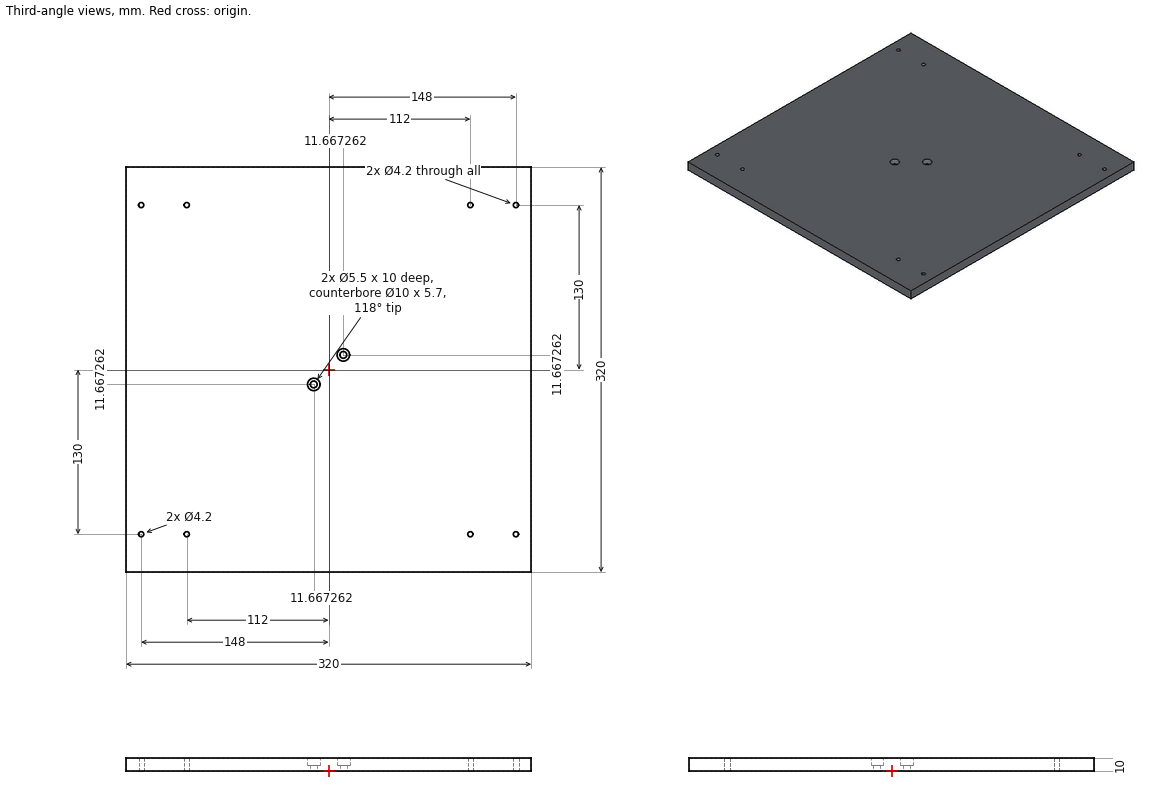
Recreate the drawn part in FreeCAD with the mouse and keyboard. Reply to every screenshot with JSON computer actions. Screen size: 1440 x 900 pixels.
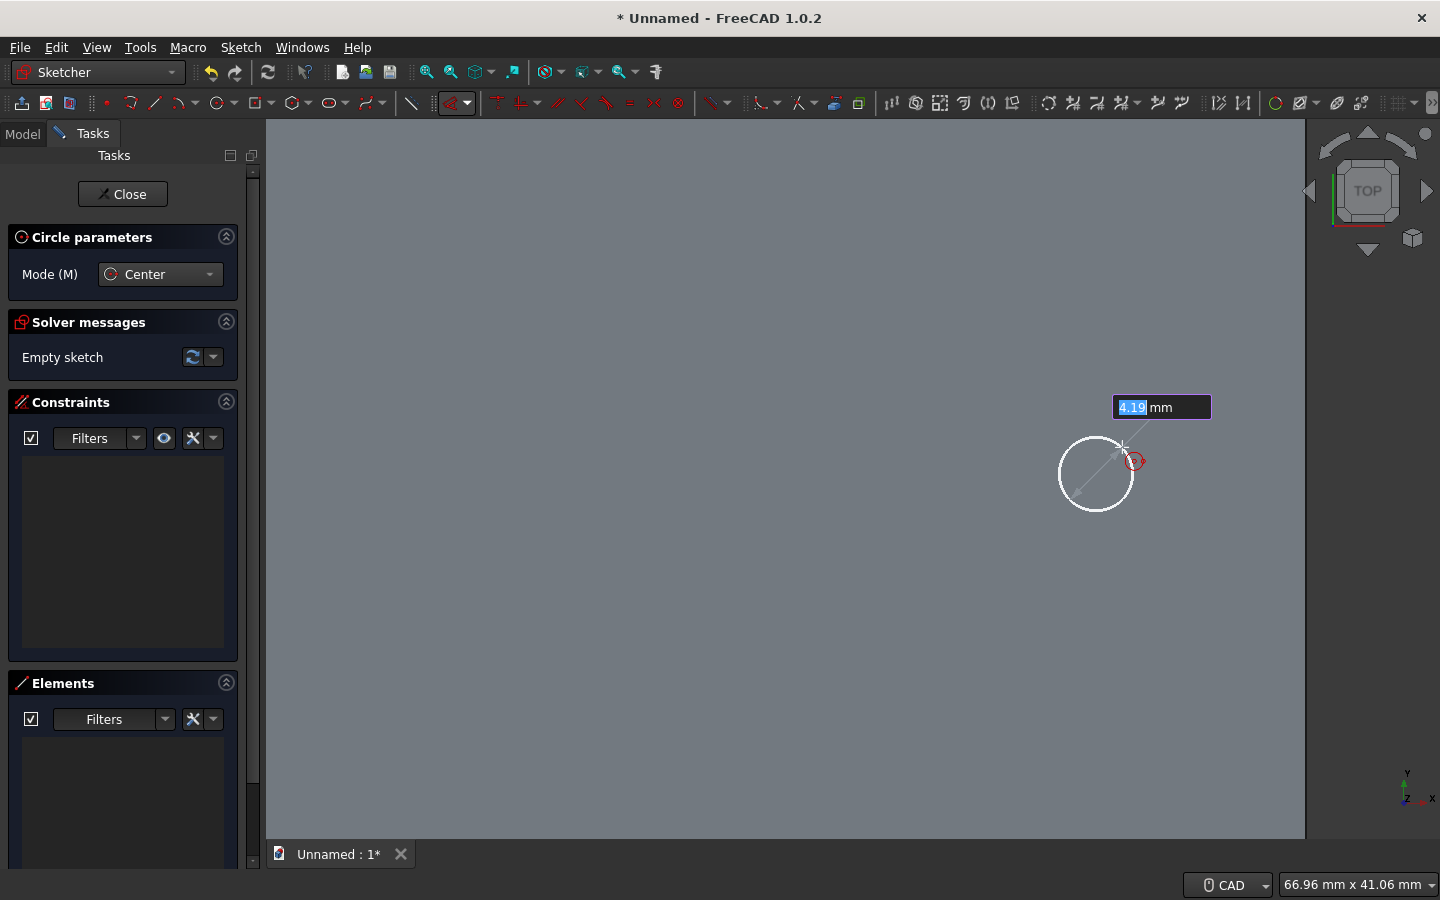
{"action": "type", "text": "4.2"}
{"action": "key", "text": "Return"}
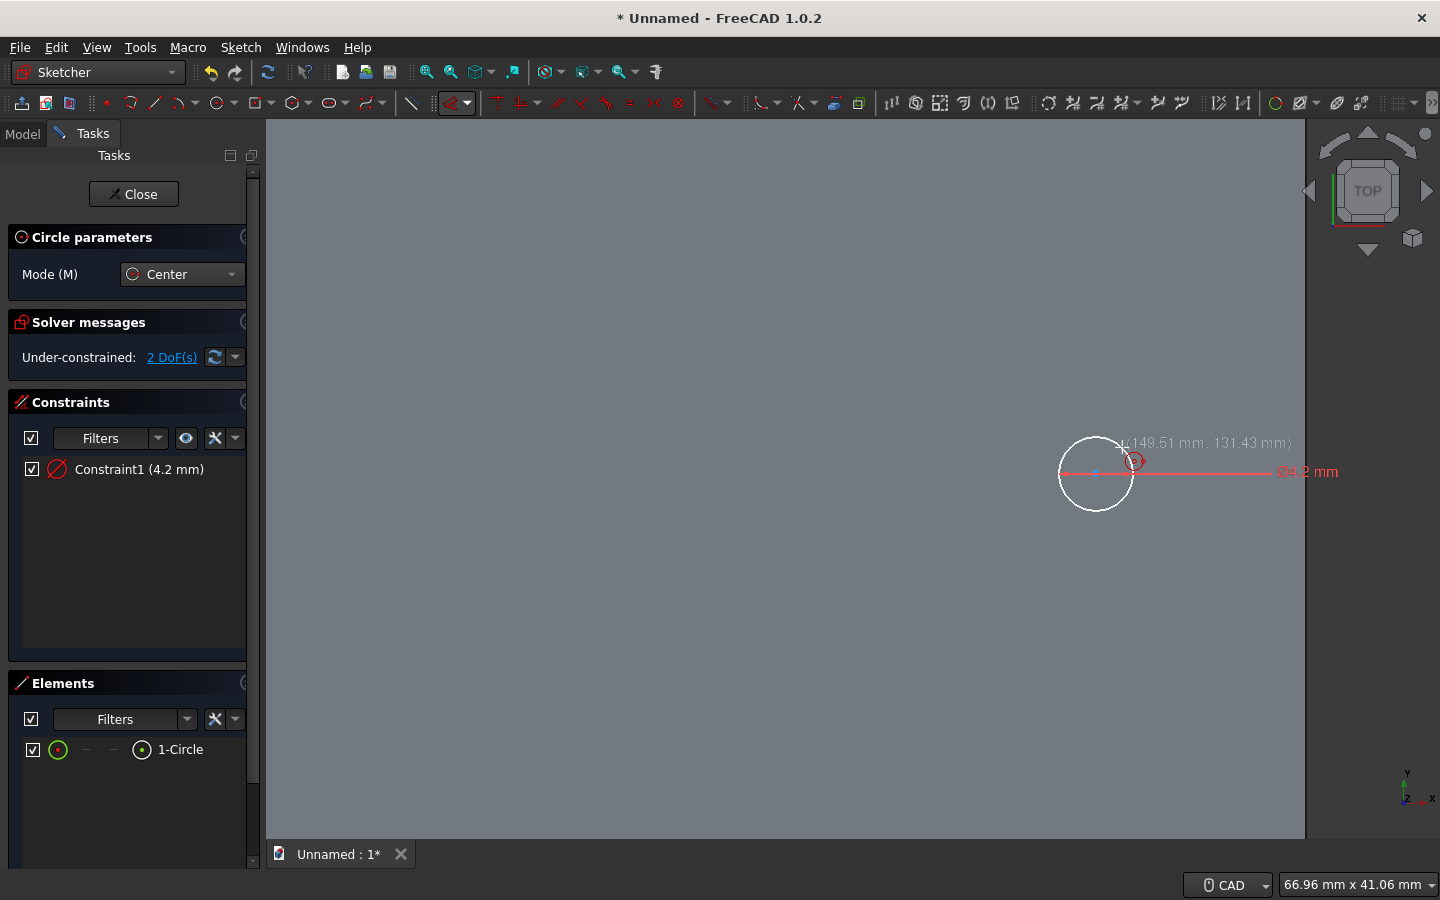
{"action": "left_click", "coordinate": [464, 473]}
{"action": "mouse_move", "coordinate": [490, 447]}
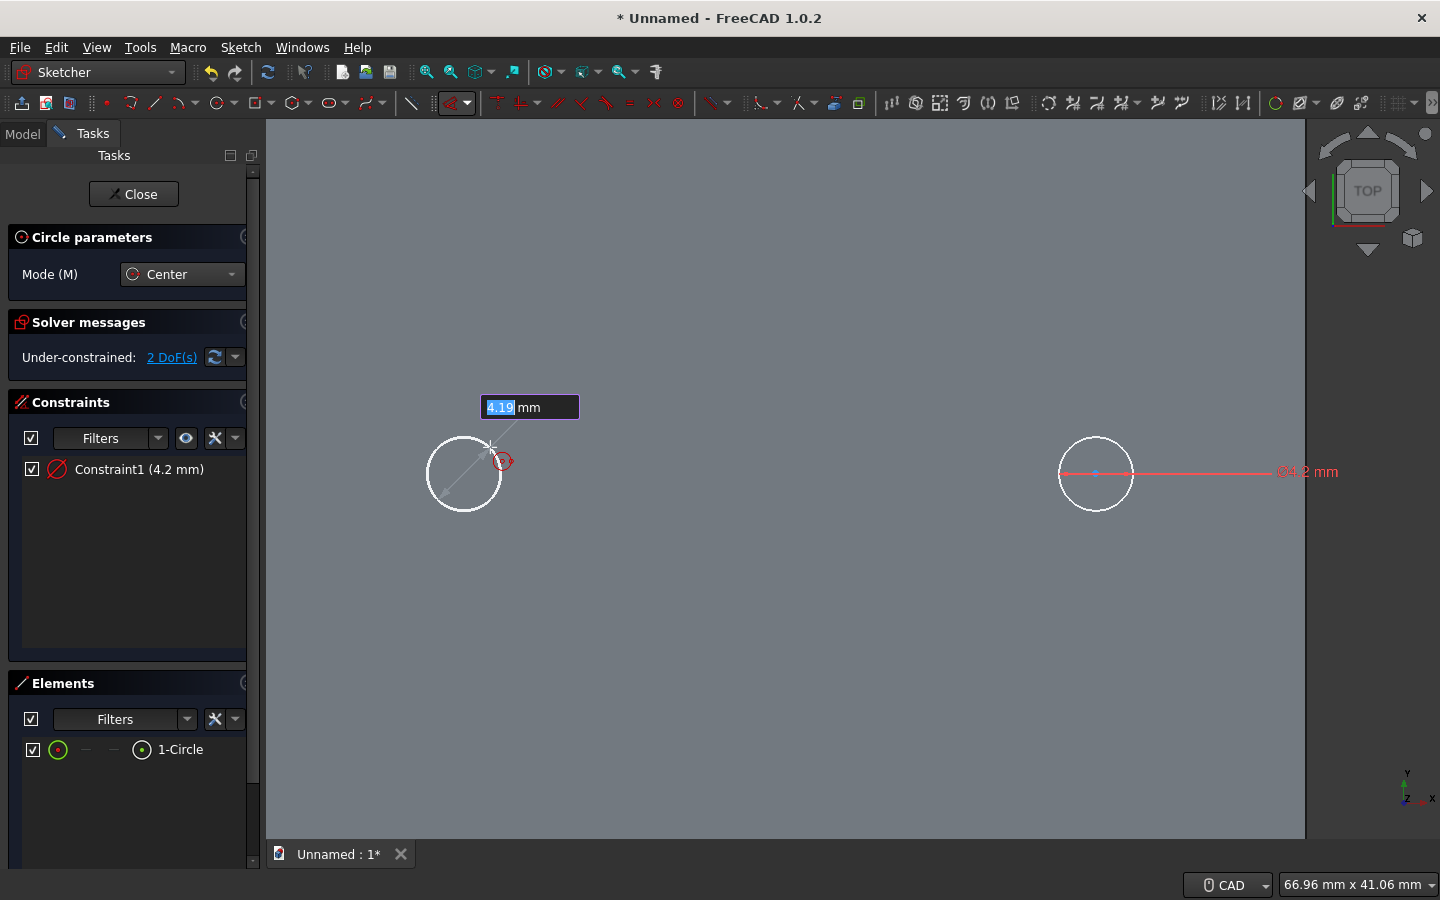
{"action": "type", "text": "4.2"}
{"action": "key", "text": "Return"}
{"action": "key", "text": "Escape"}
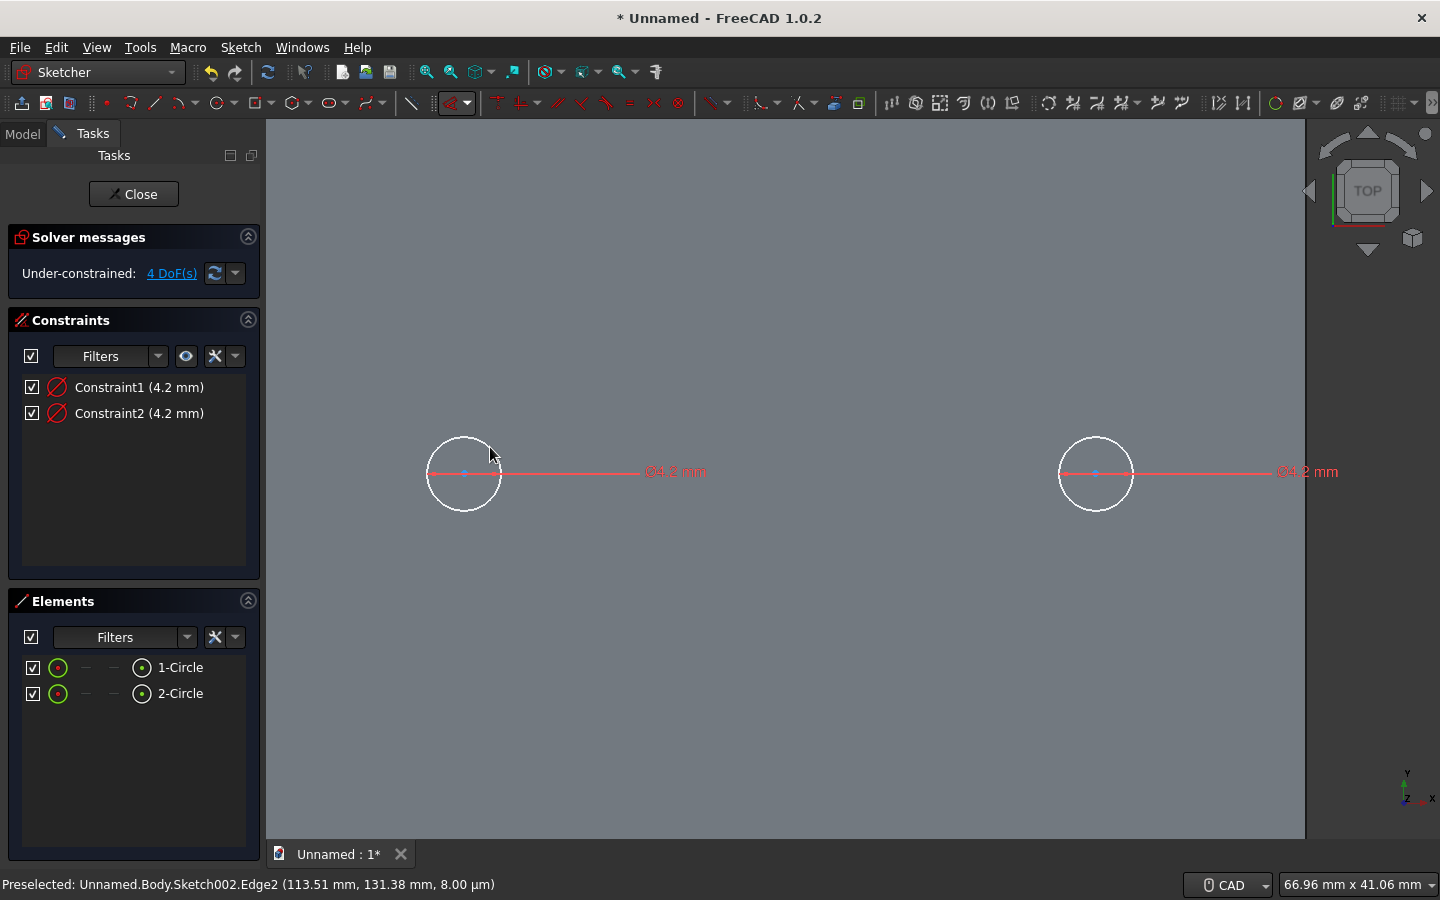
{"action": "left_click", "coordinate": [450, 104]}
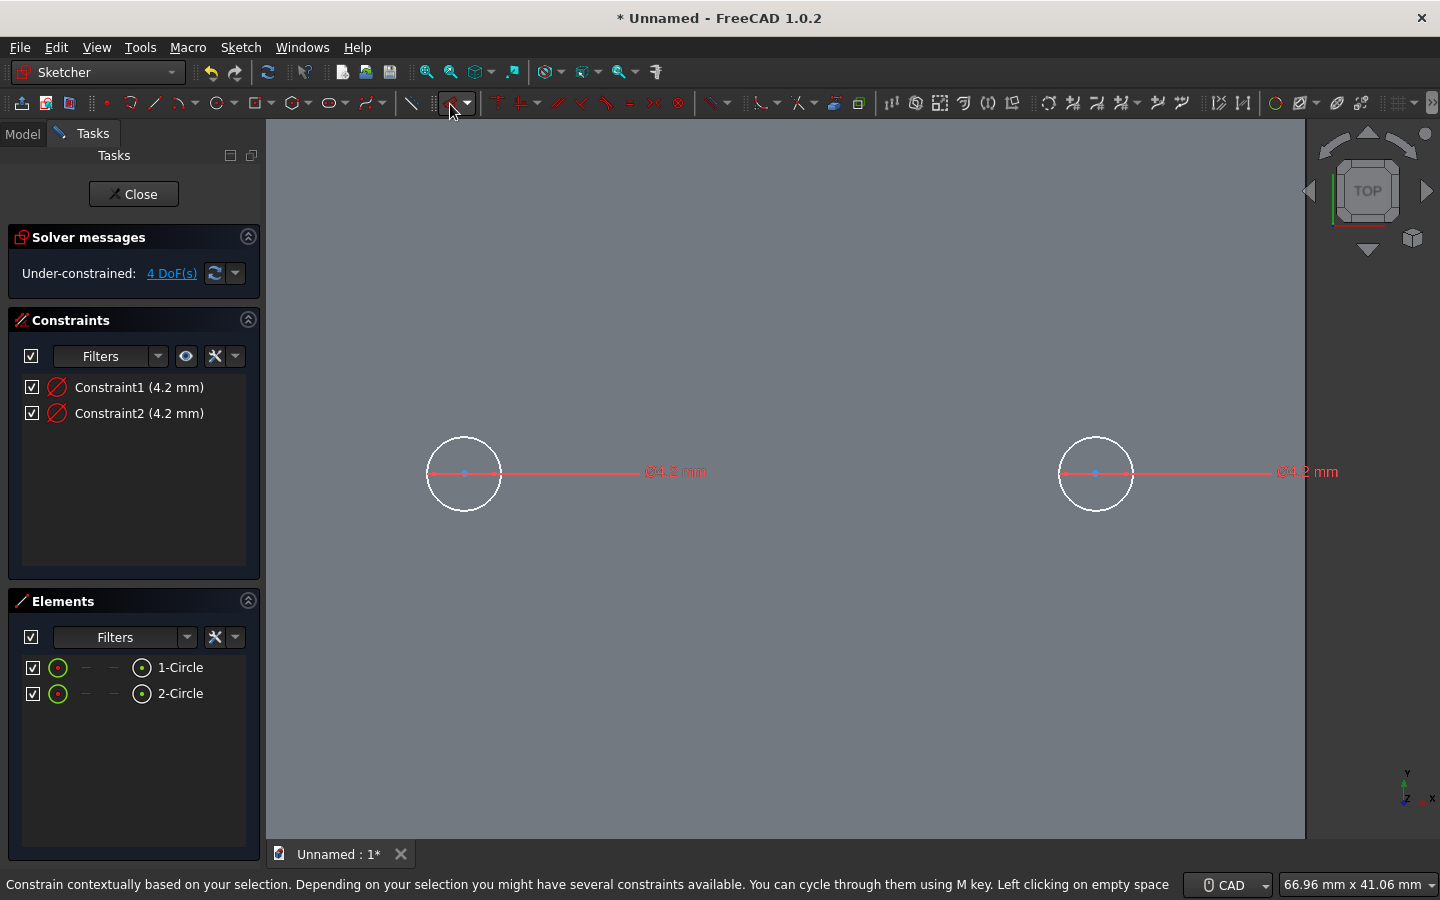
{"action": "left_click", "coordinate": [1096, 474]}
{"action": "left_click", "coordinate": [695, 440]}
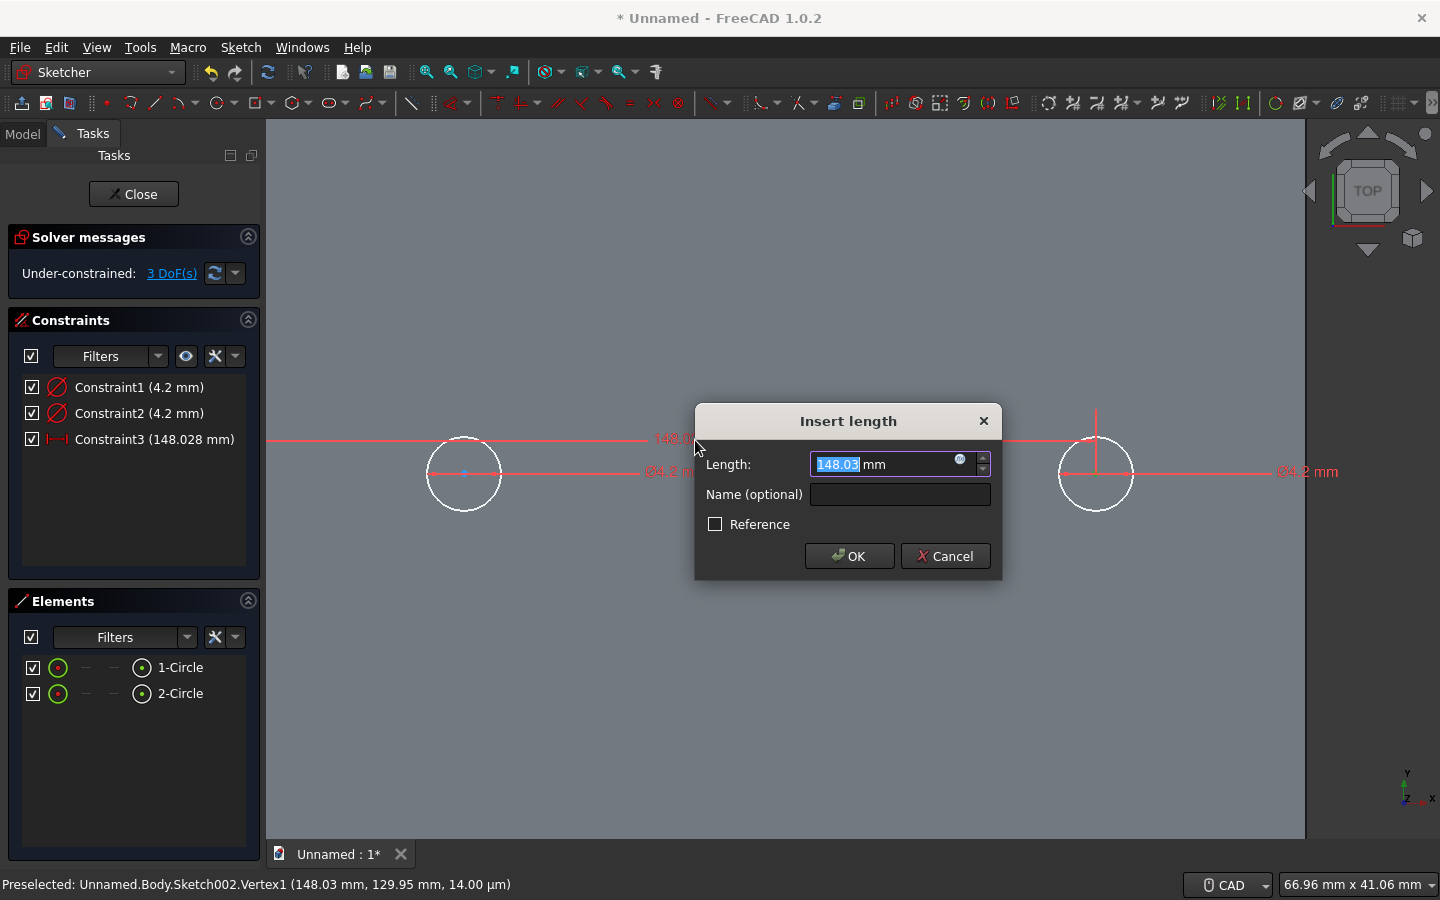
{"action": "type", "text": "148"}
{"action": "key", "text": "Return"}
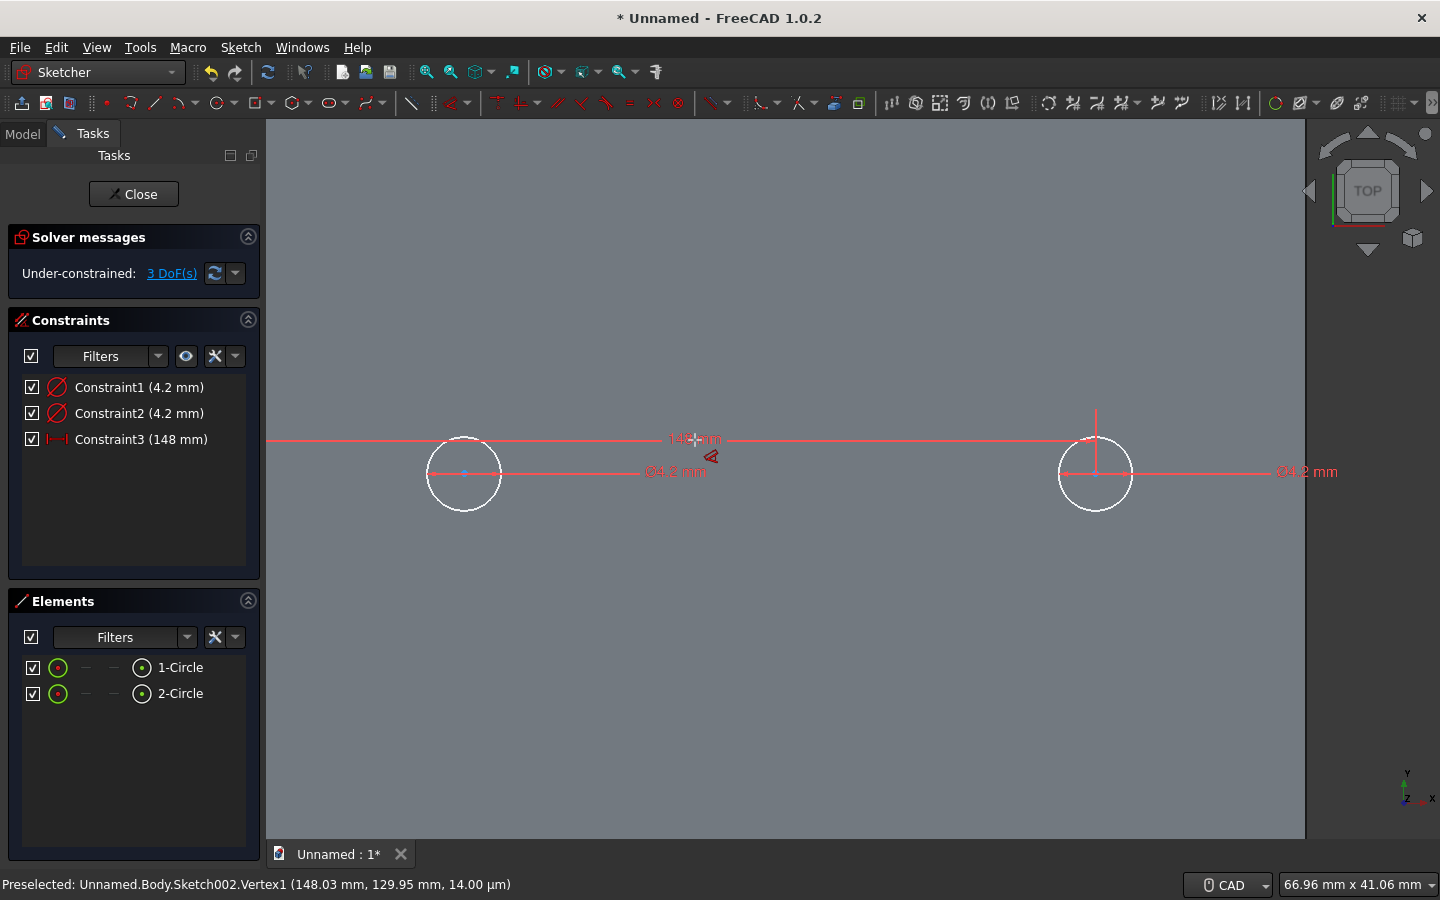
{"action": "left_click", "coordinate": [1096, 474]}
{"action": "left_click", "coordinate": [1130, 642]}